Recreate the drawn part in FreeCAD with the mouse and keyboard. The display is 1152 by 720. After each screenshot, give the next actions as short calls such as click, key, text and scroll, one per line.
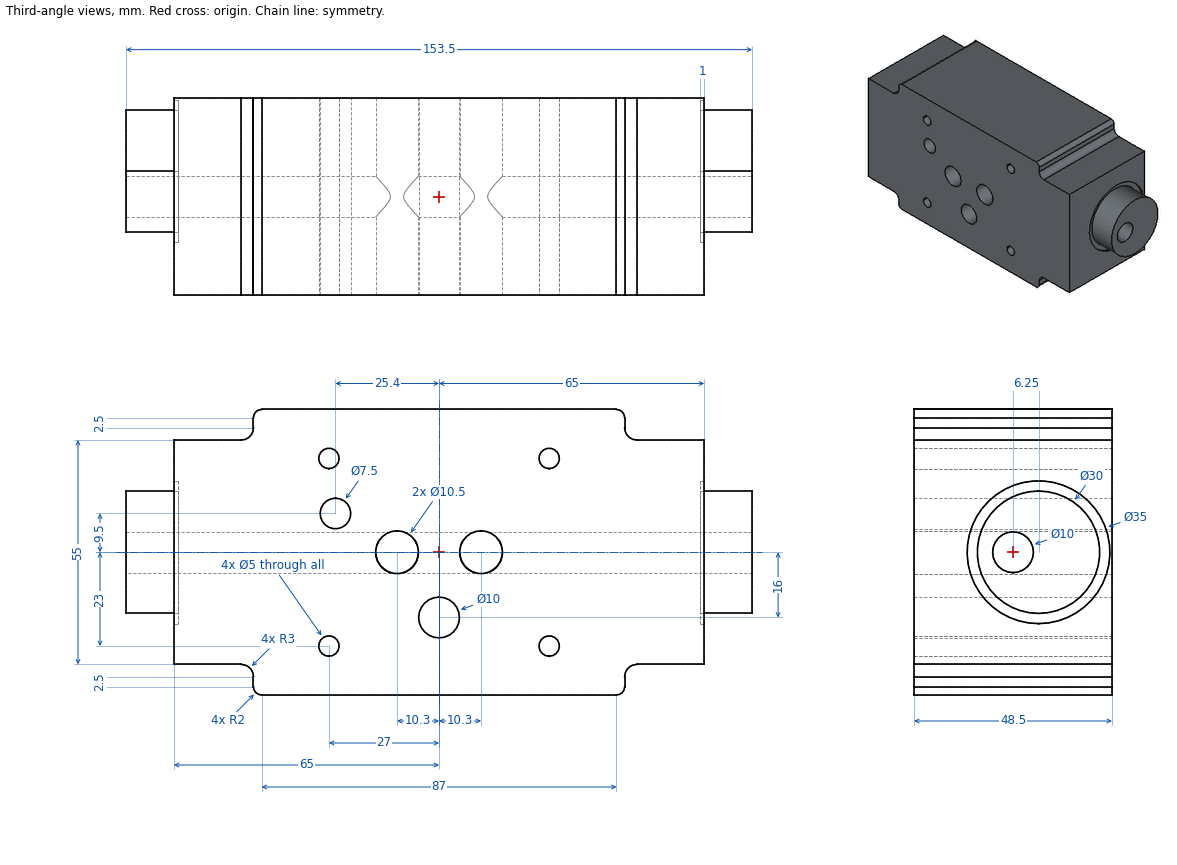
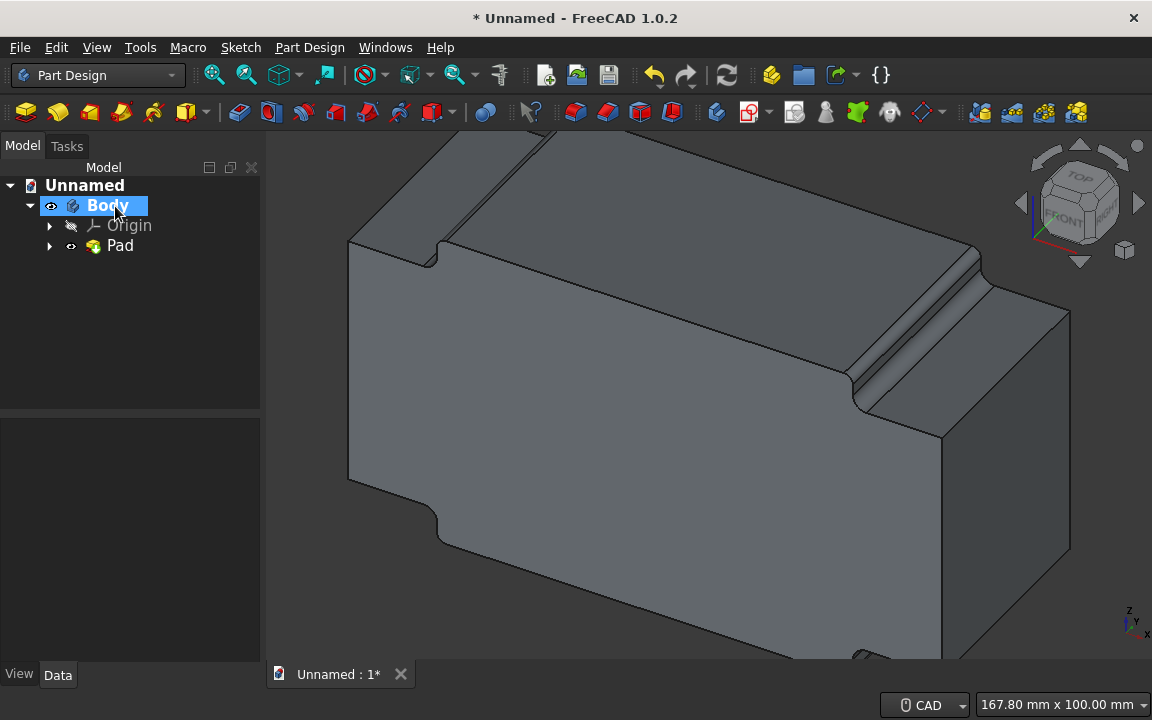
click(216, 76)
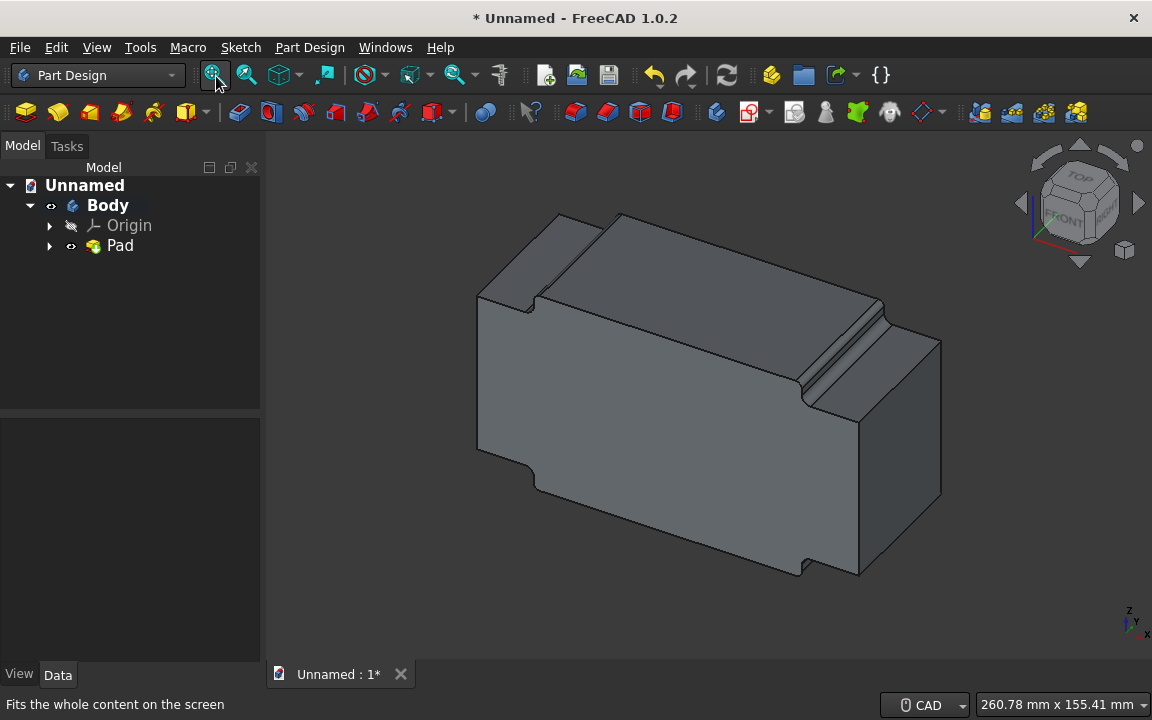
click(900, 457)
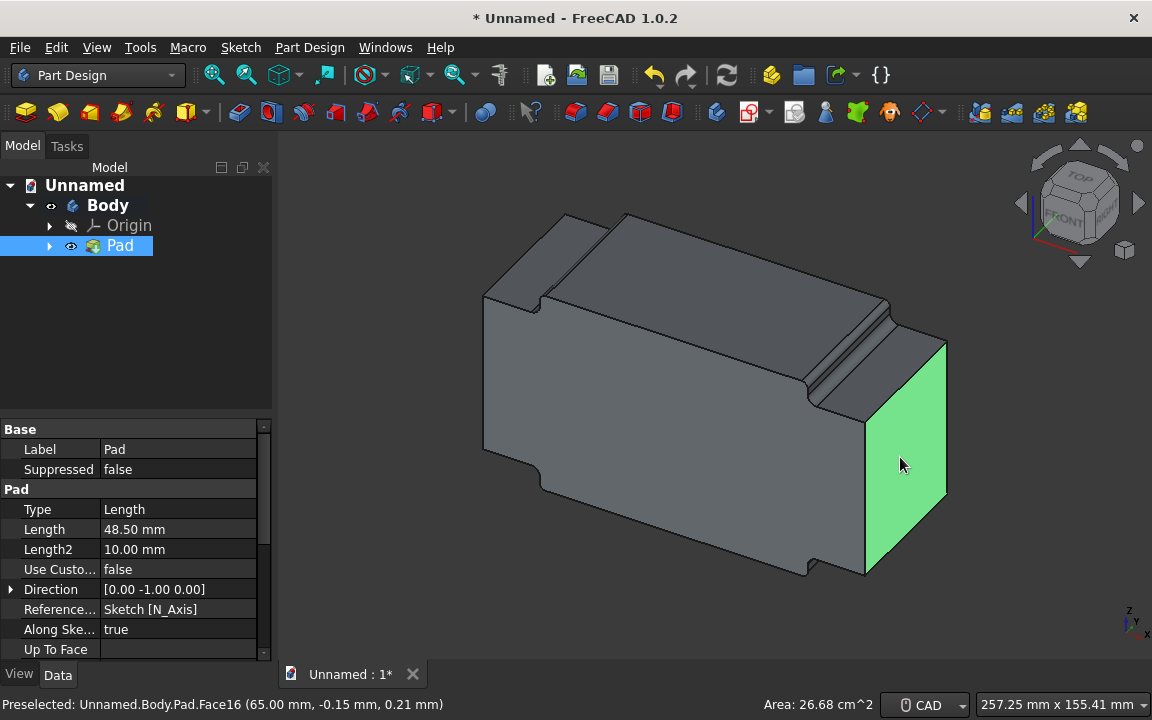
click(750, 112)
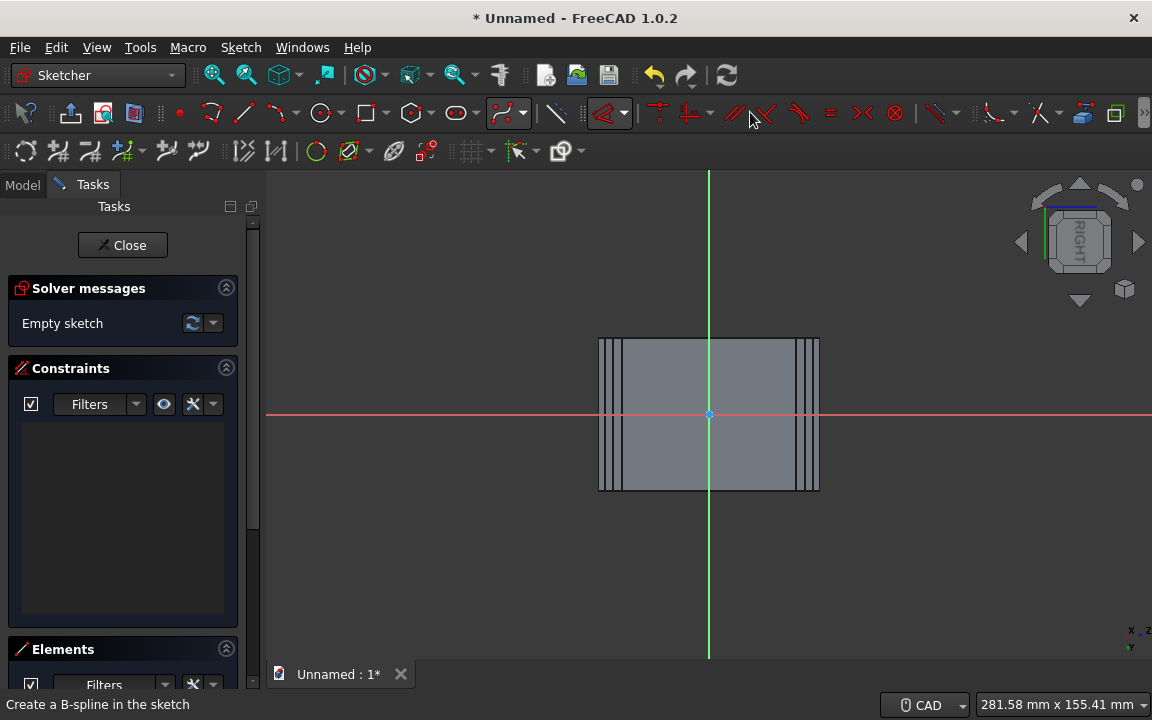
scroll(749, 446, up, 5)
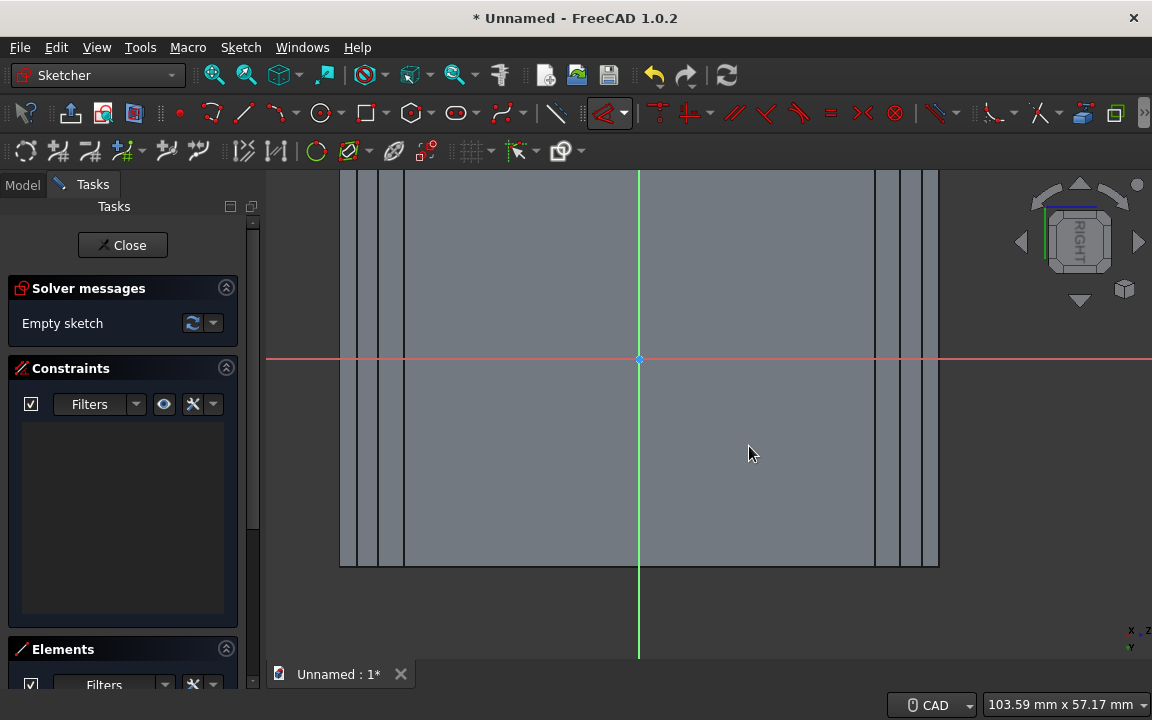
click(322, 114)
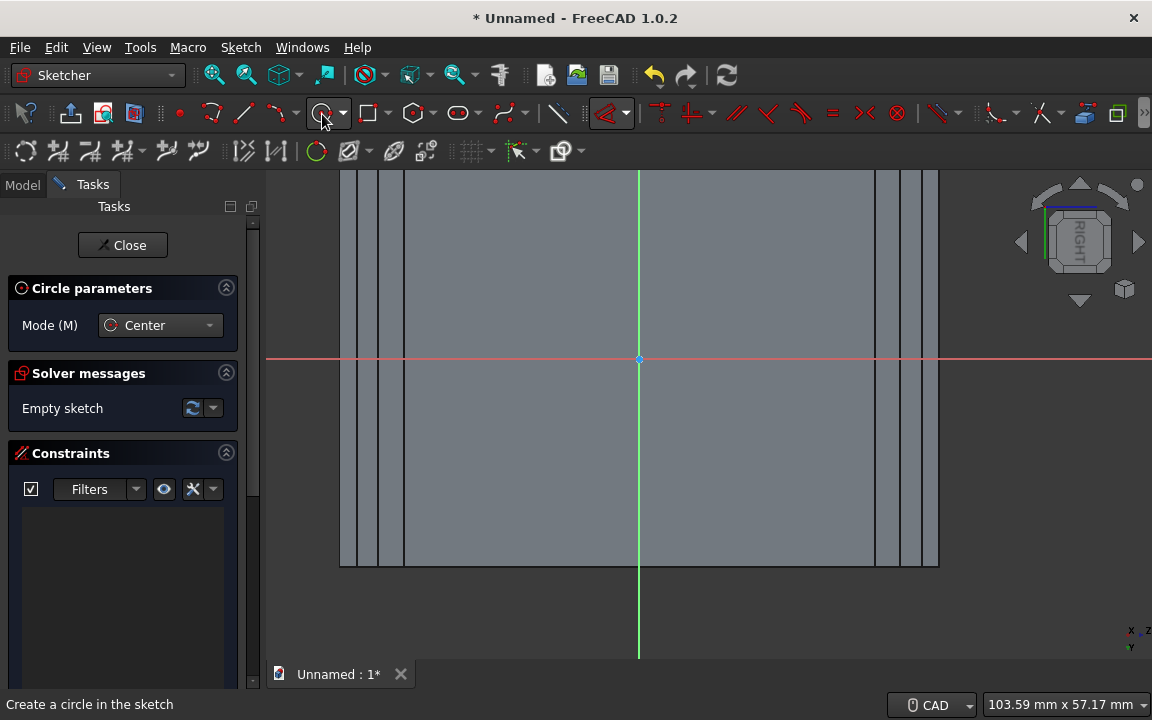
click(639, 413)
move(745, 307)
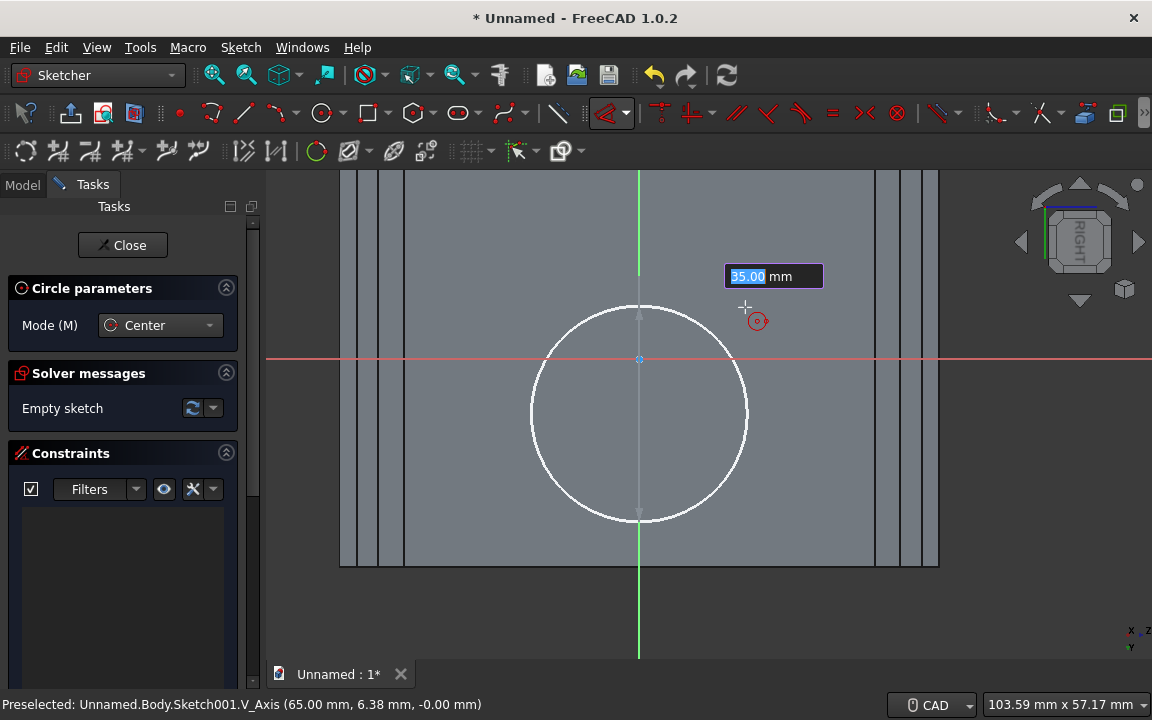
text(35)
key(Return)
key(Escape)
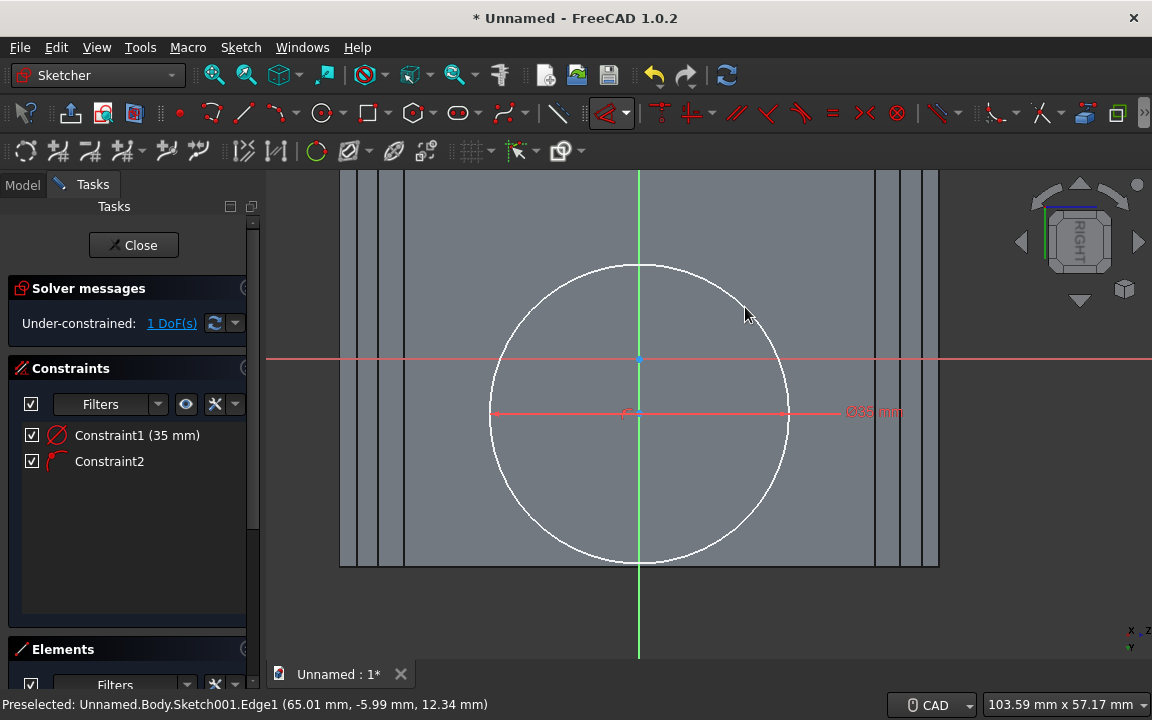
click(639, 414)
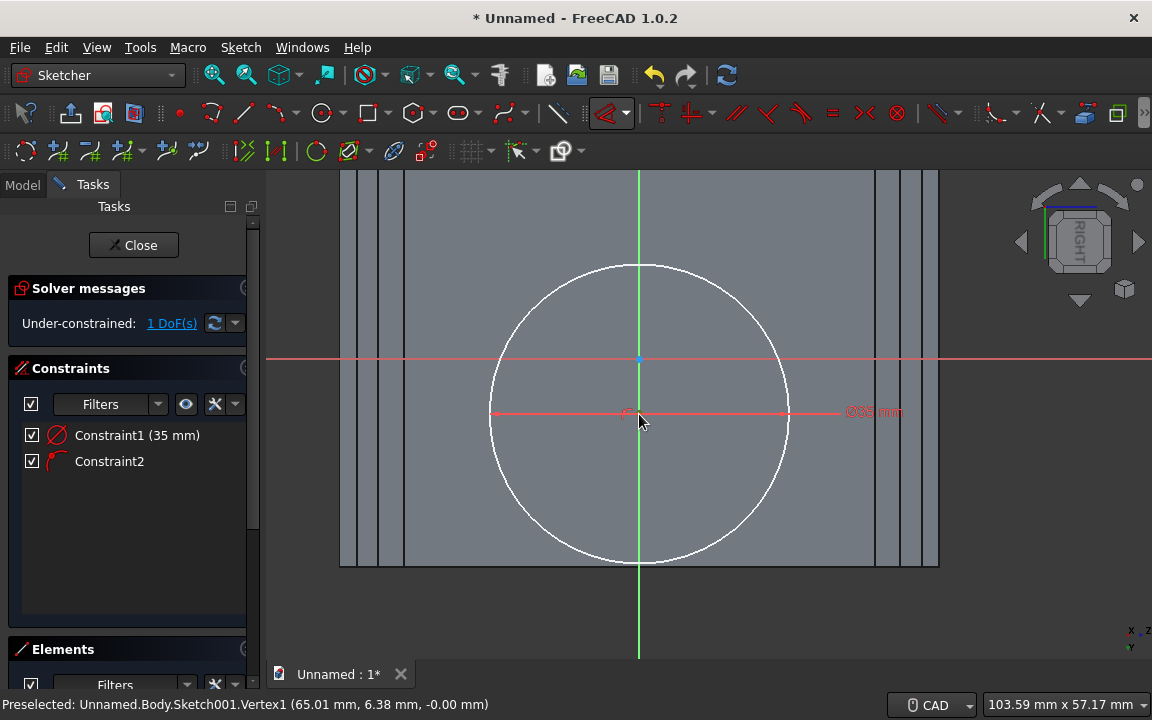
click(628, 114)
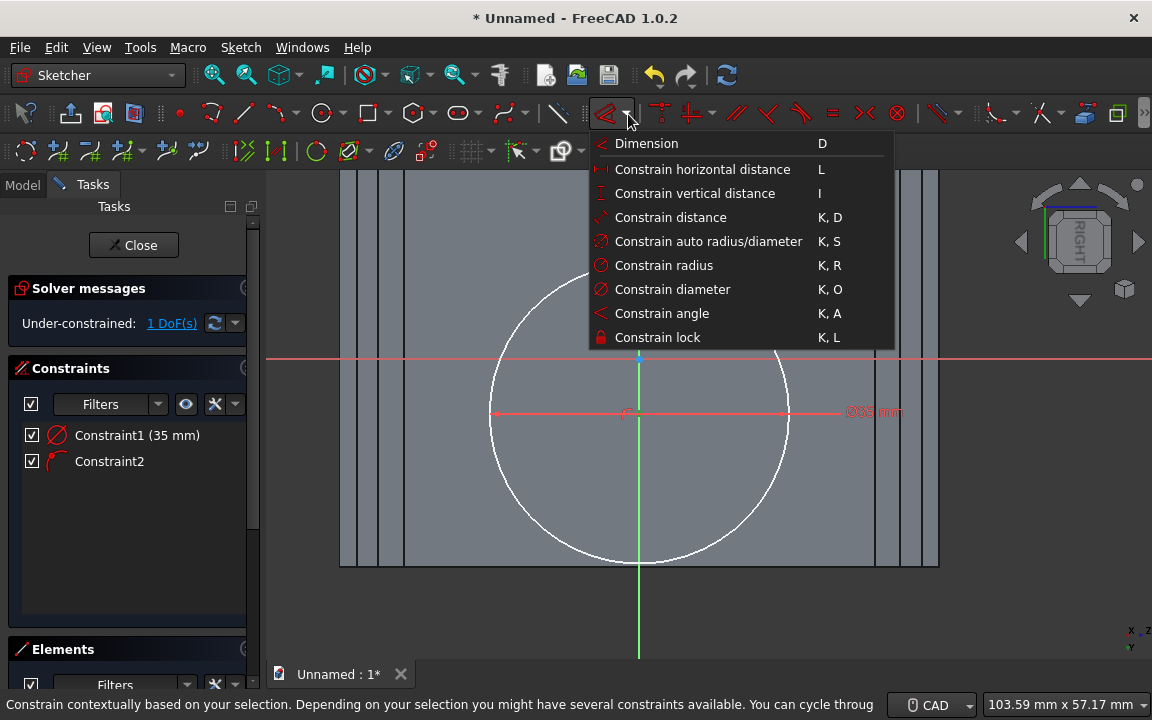
click(742, 193)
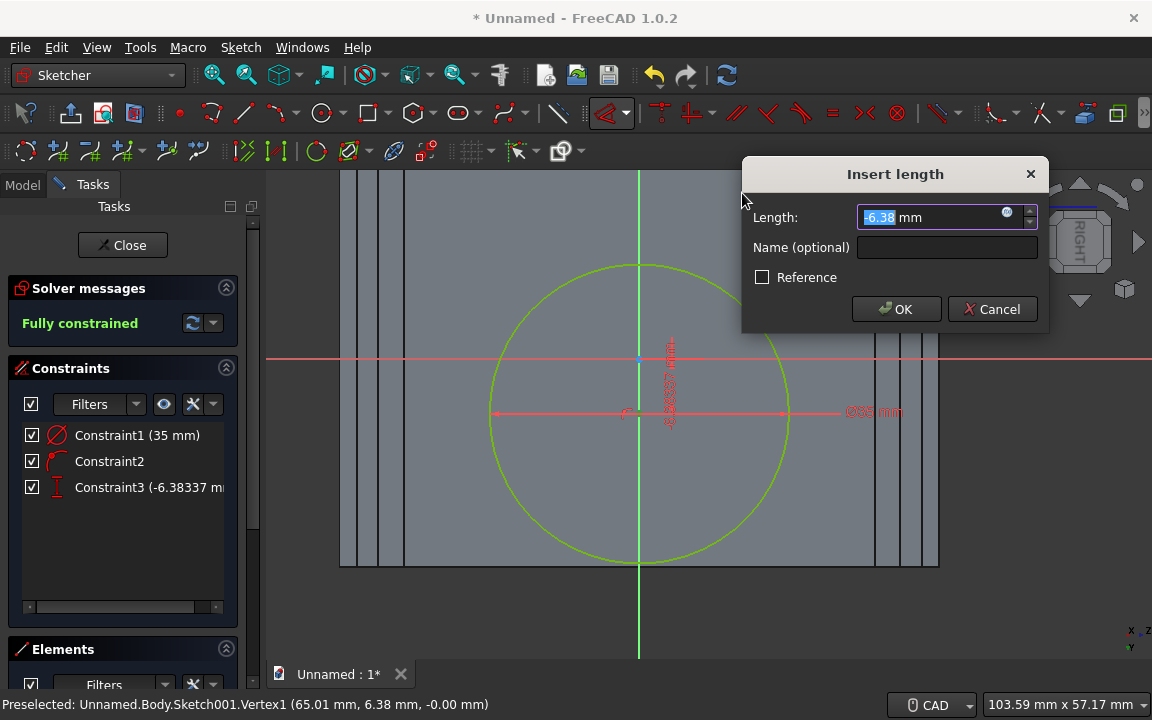
text(-6.25)
key(Return)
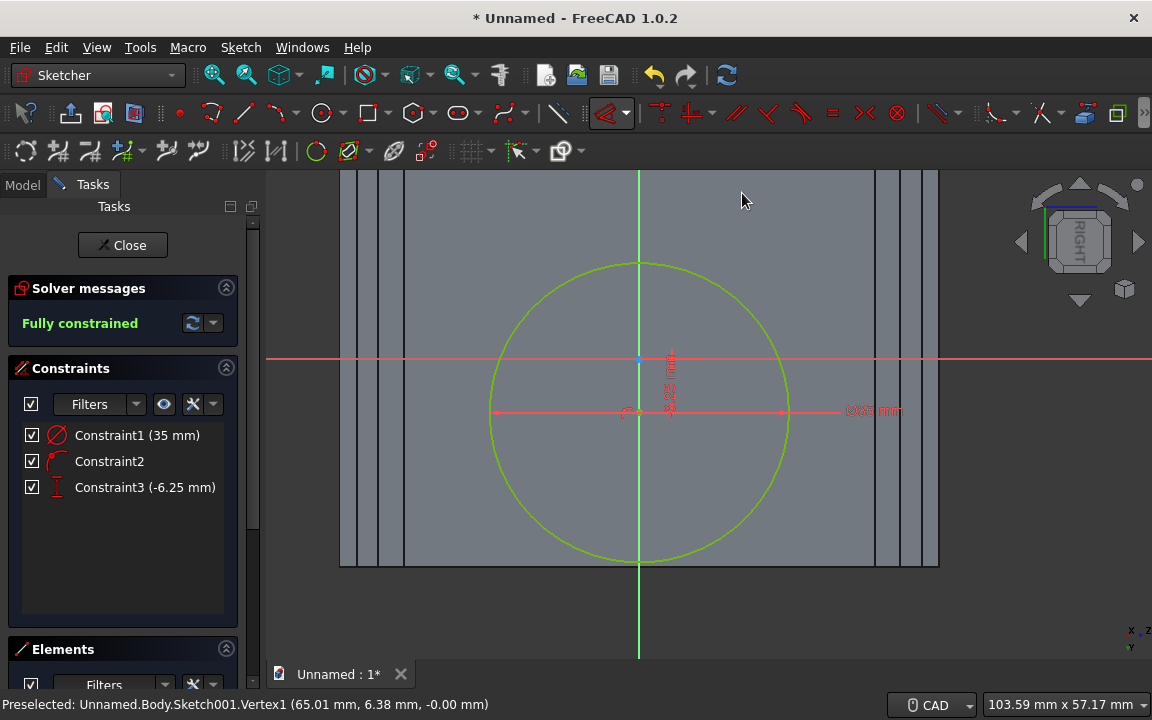
click(123, 245)